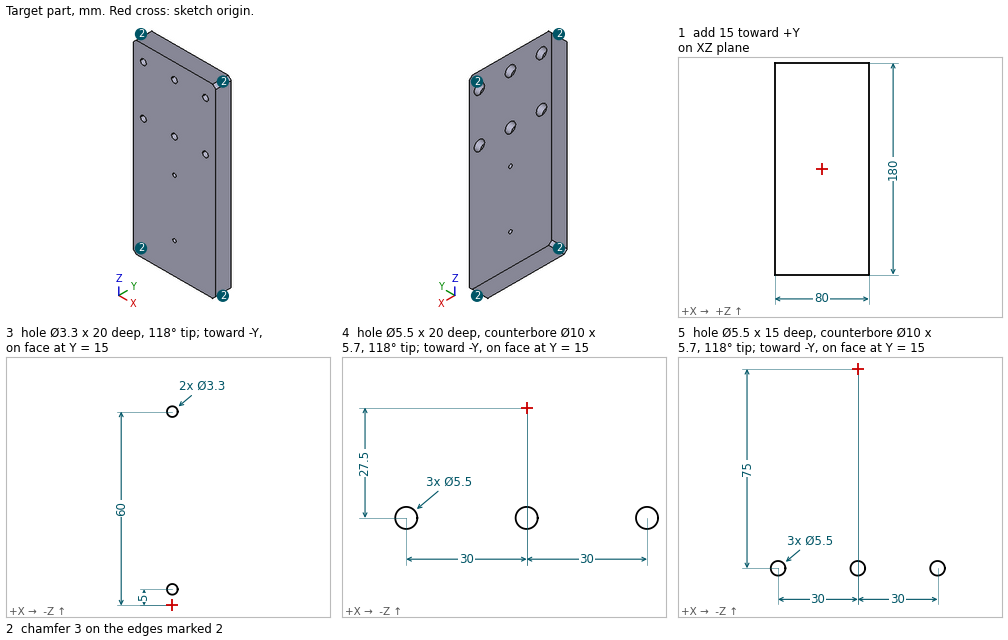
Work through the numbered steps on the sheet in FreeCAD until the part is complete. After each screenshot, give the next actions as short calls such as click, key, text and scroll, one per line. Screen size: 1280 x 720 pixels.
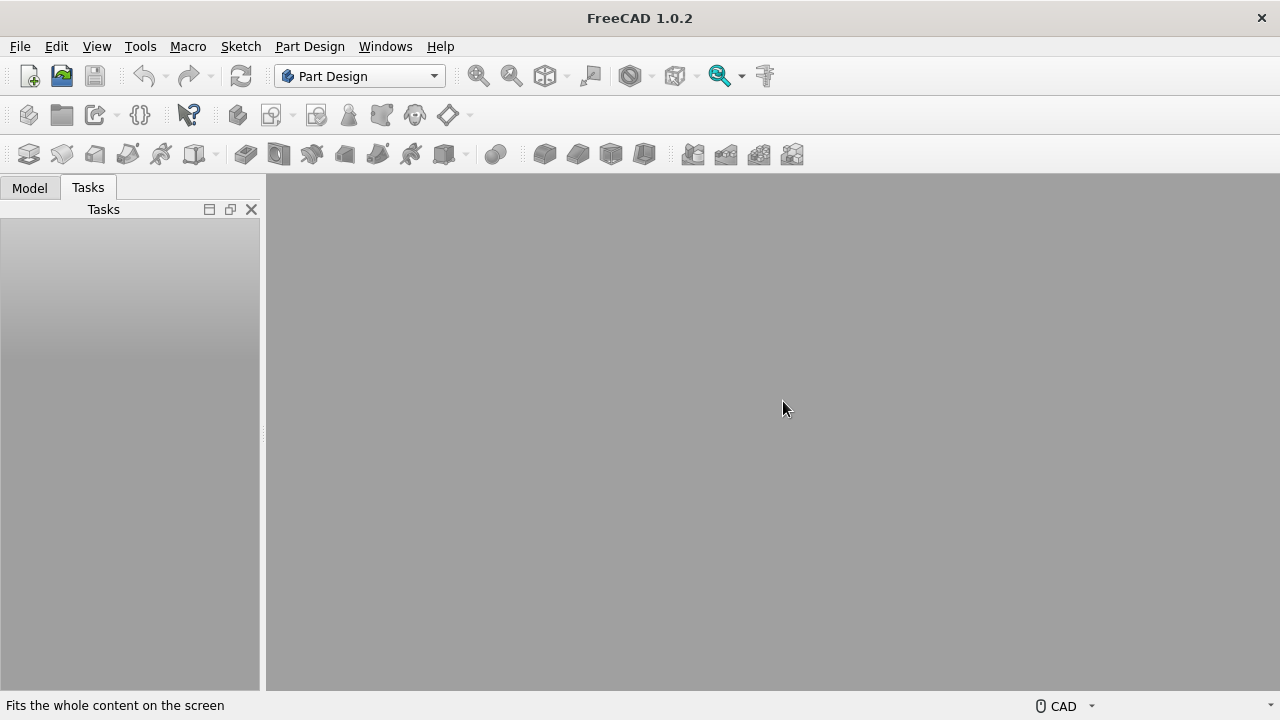
click(29, 76)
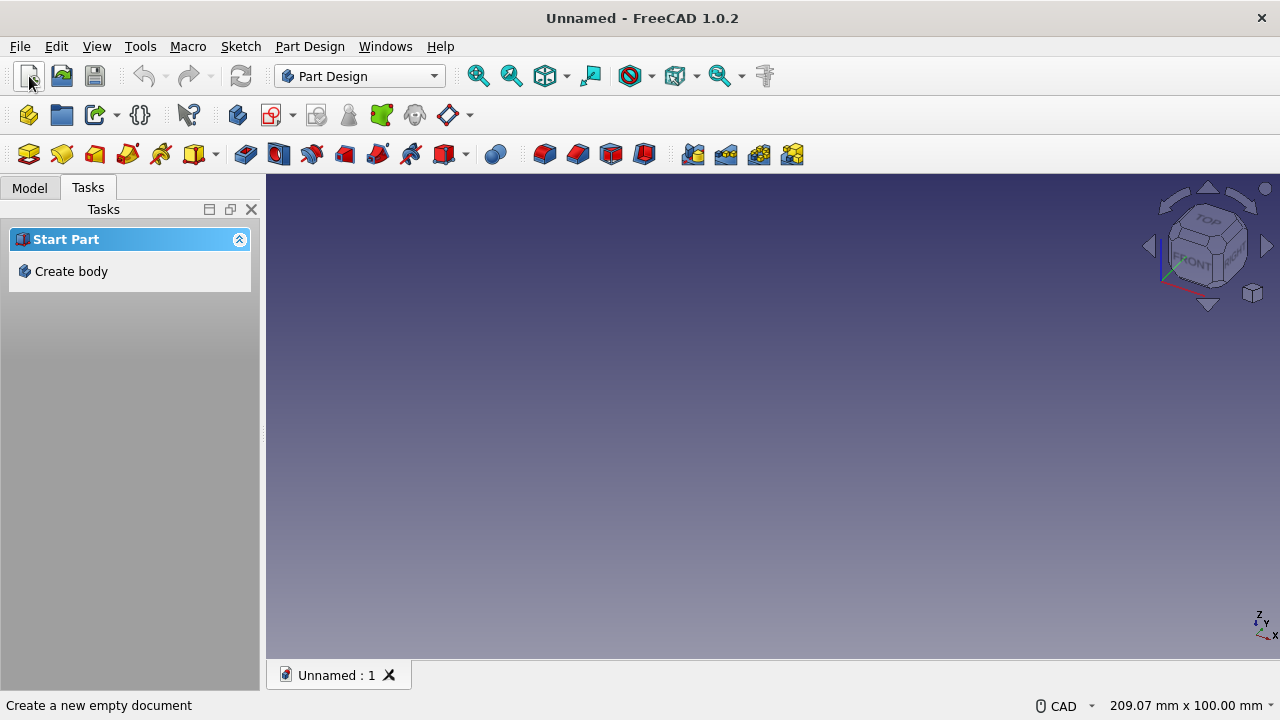
click(270, 116)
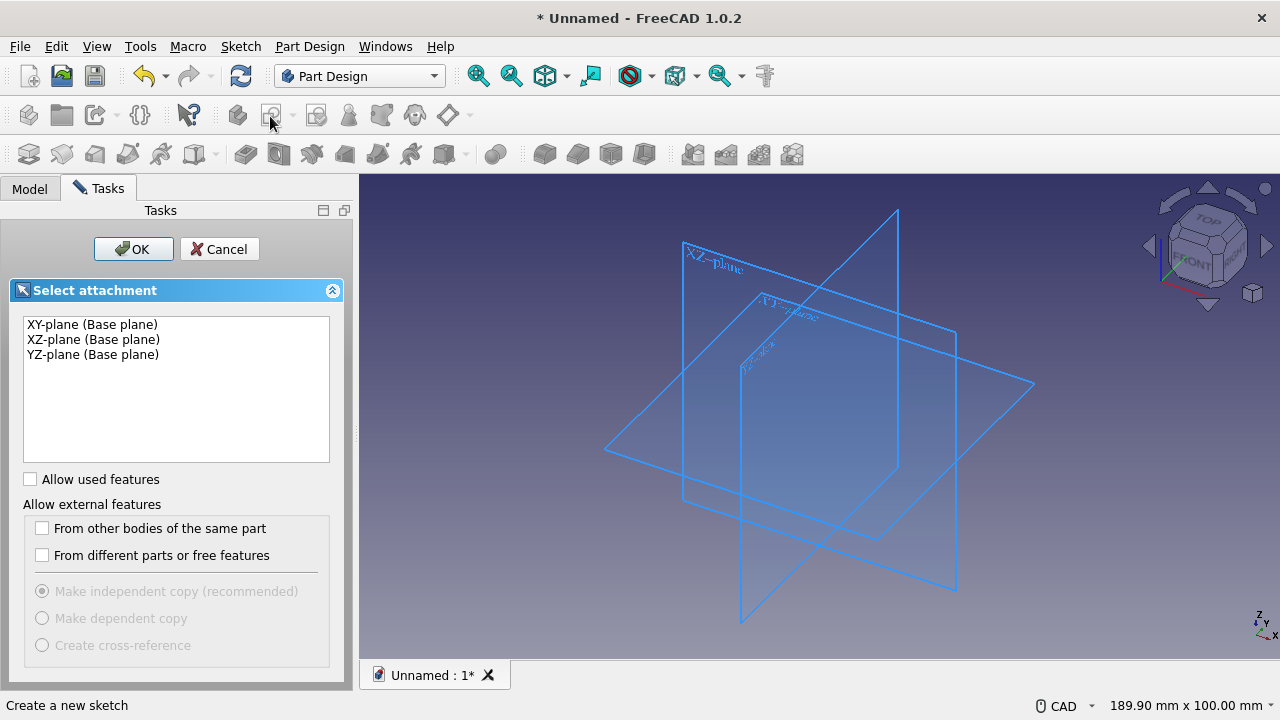
click(84, 340)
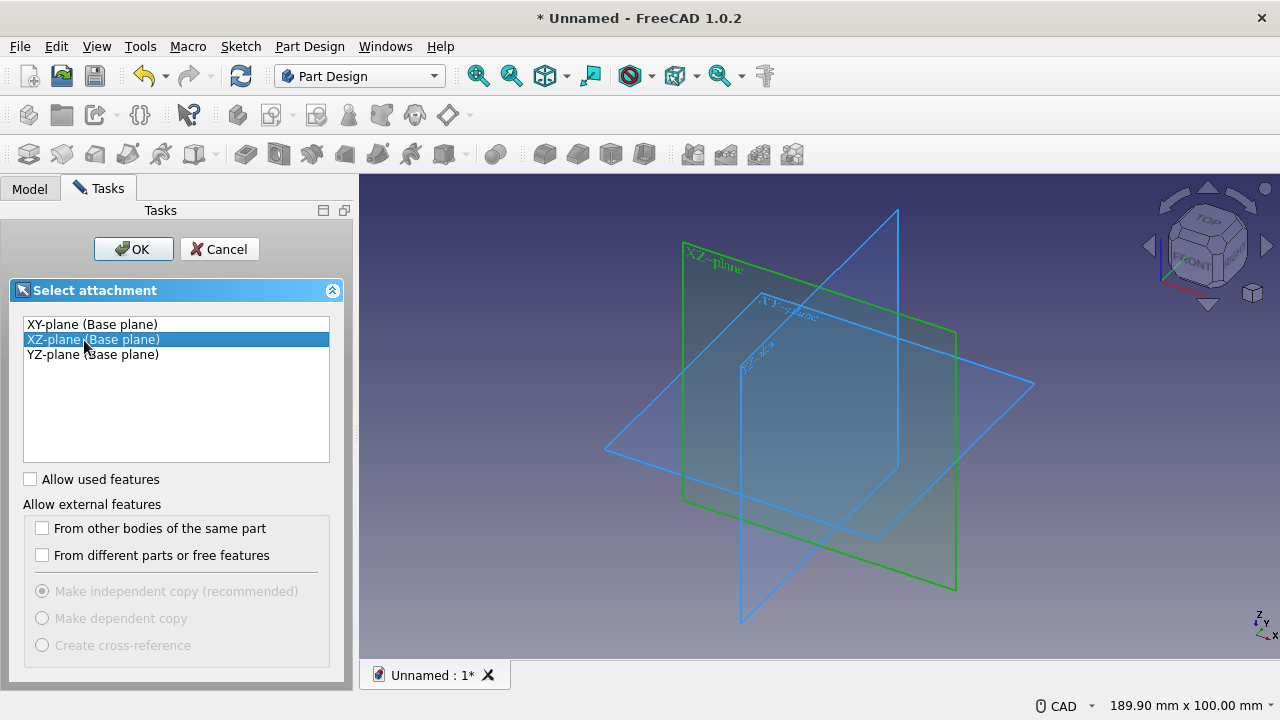
click(134, 249)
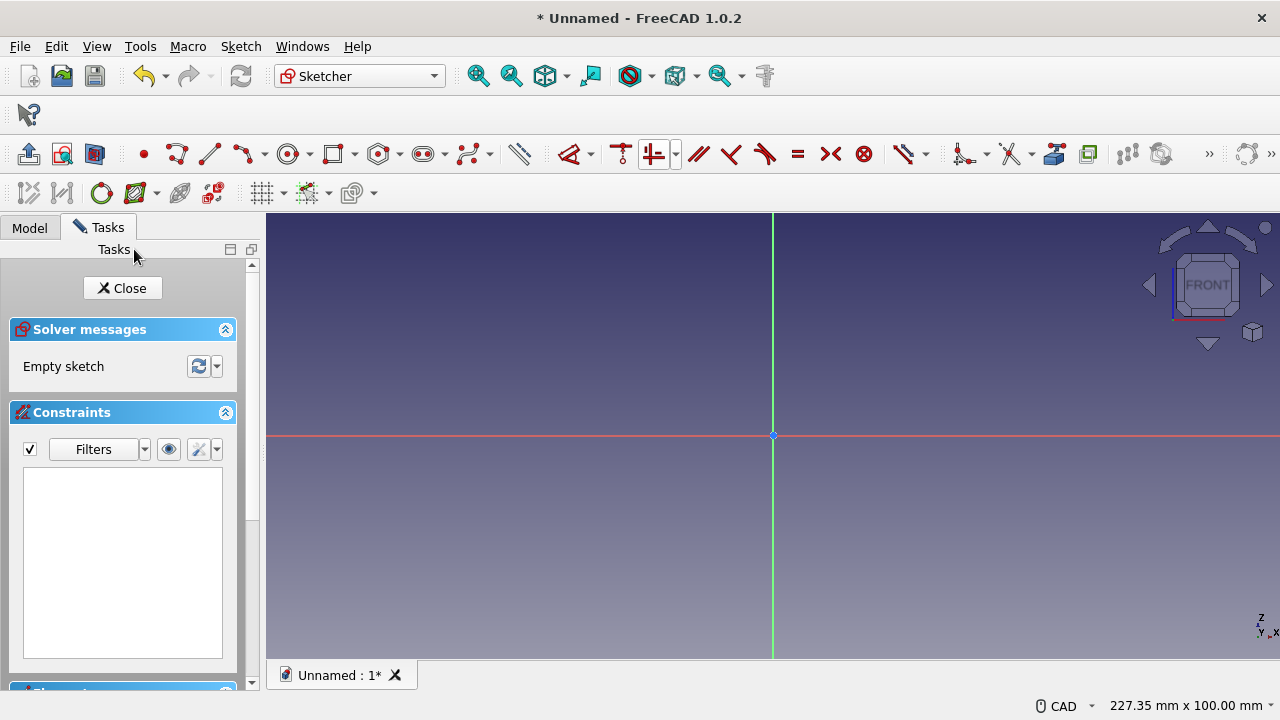
scroll(665, 436, down, 5)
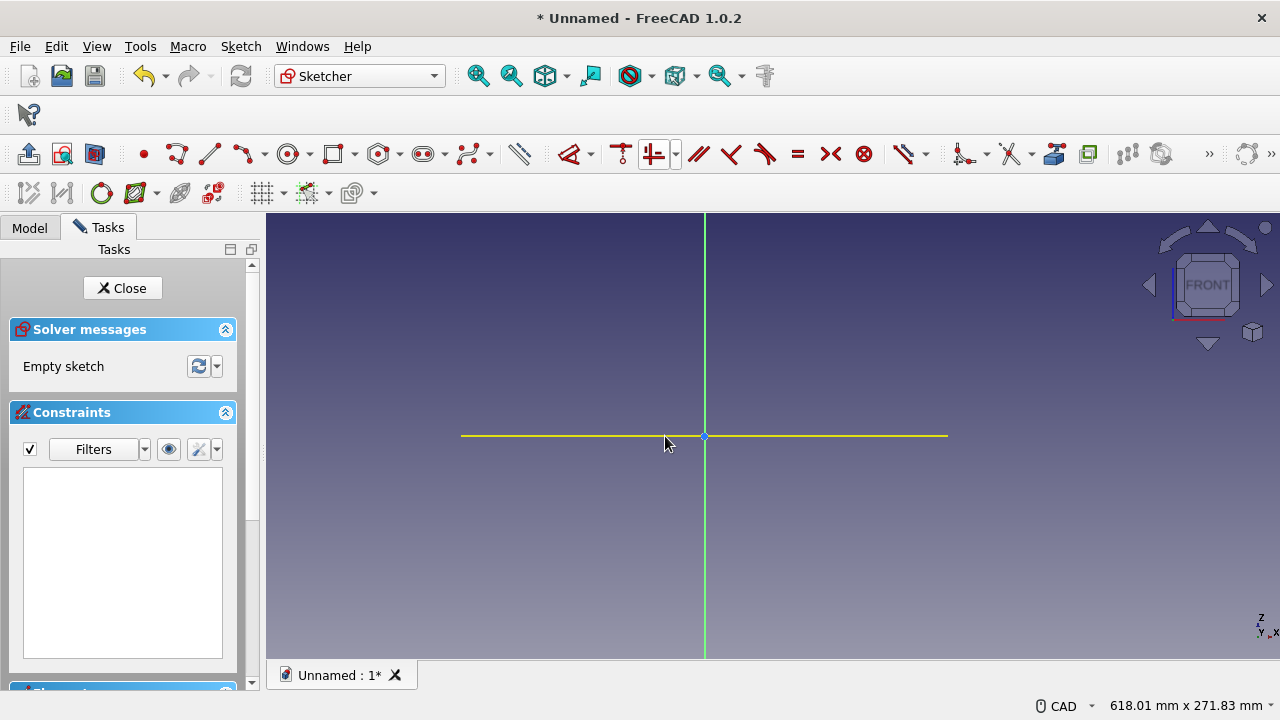
click(354, 154)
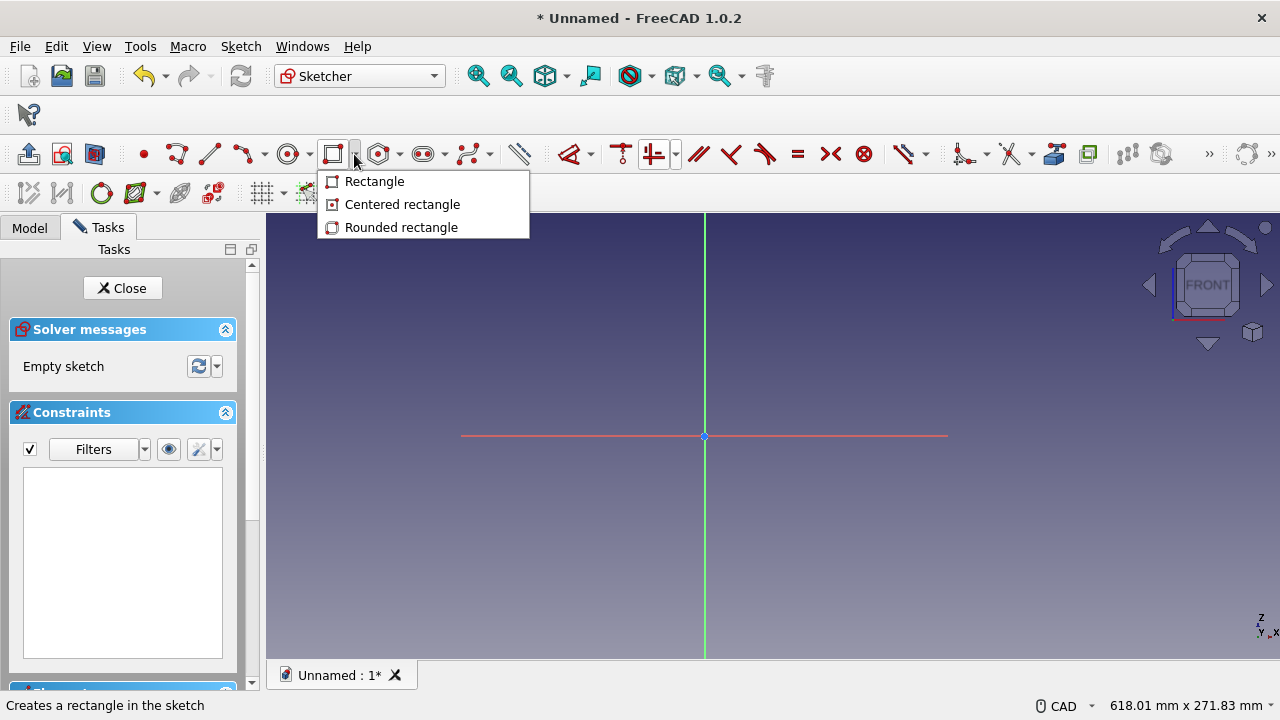
click(424, 204)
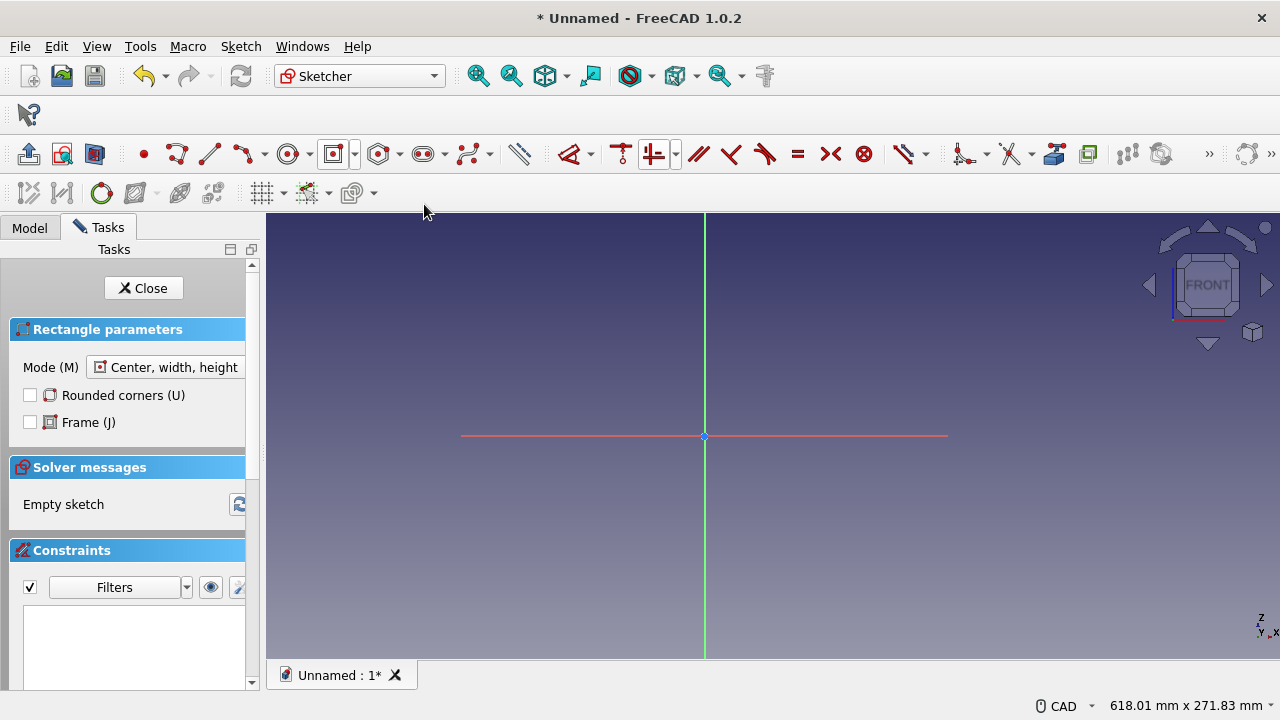
click(705, 436)
click(771, 289)
key(Escape)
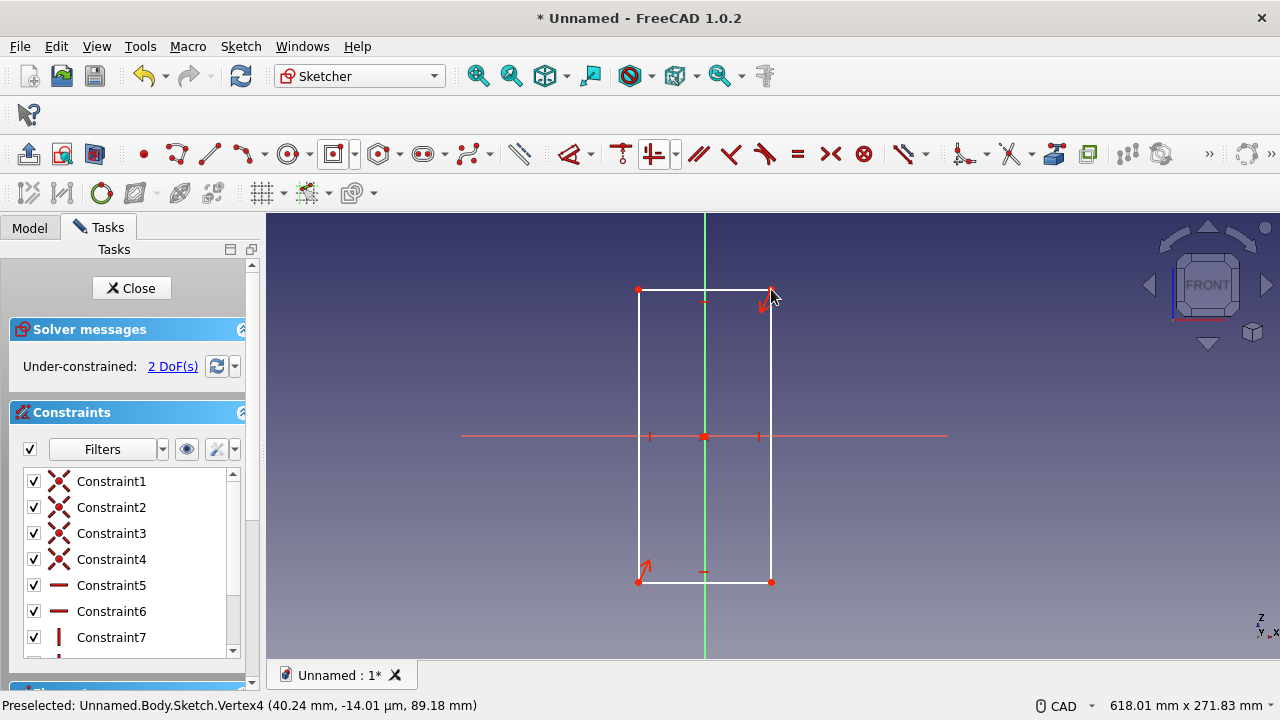
click(568, 154)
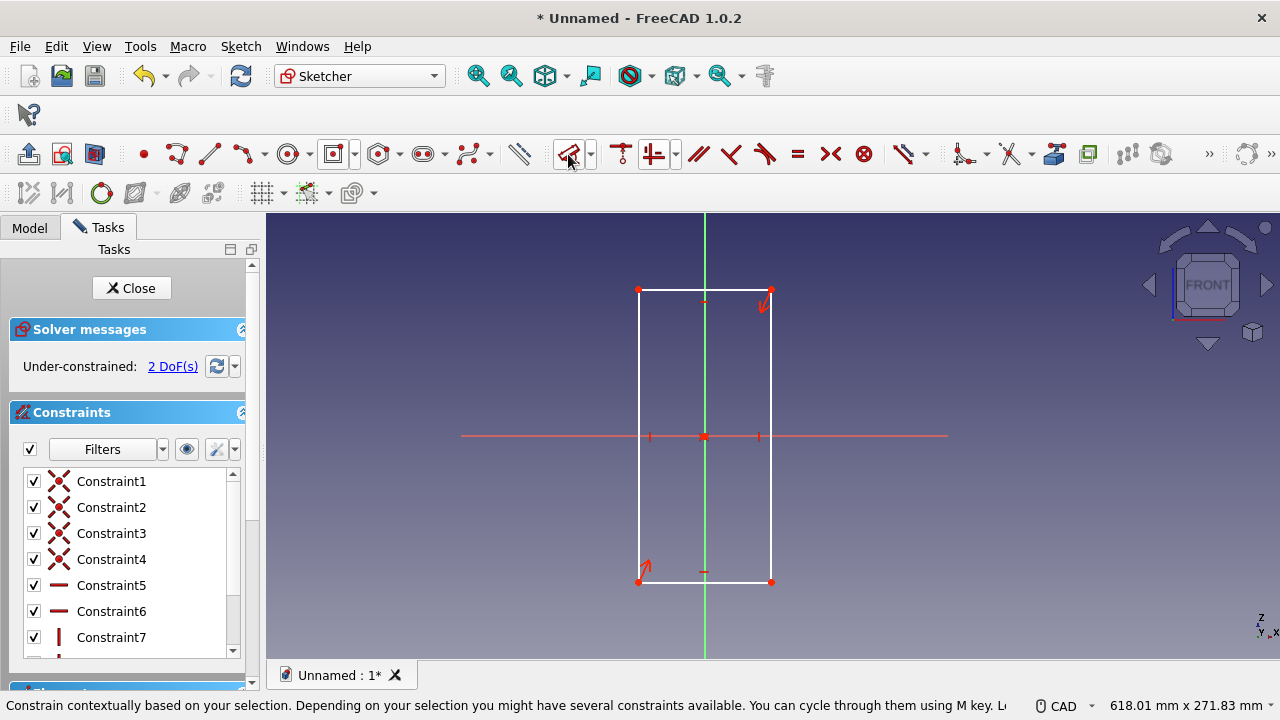
click(679, 583)
click(675, 617)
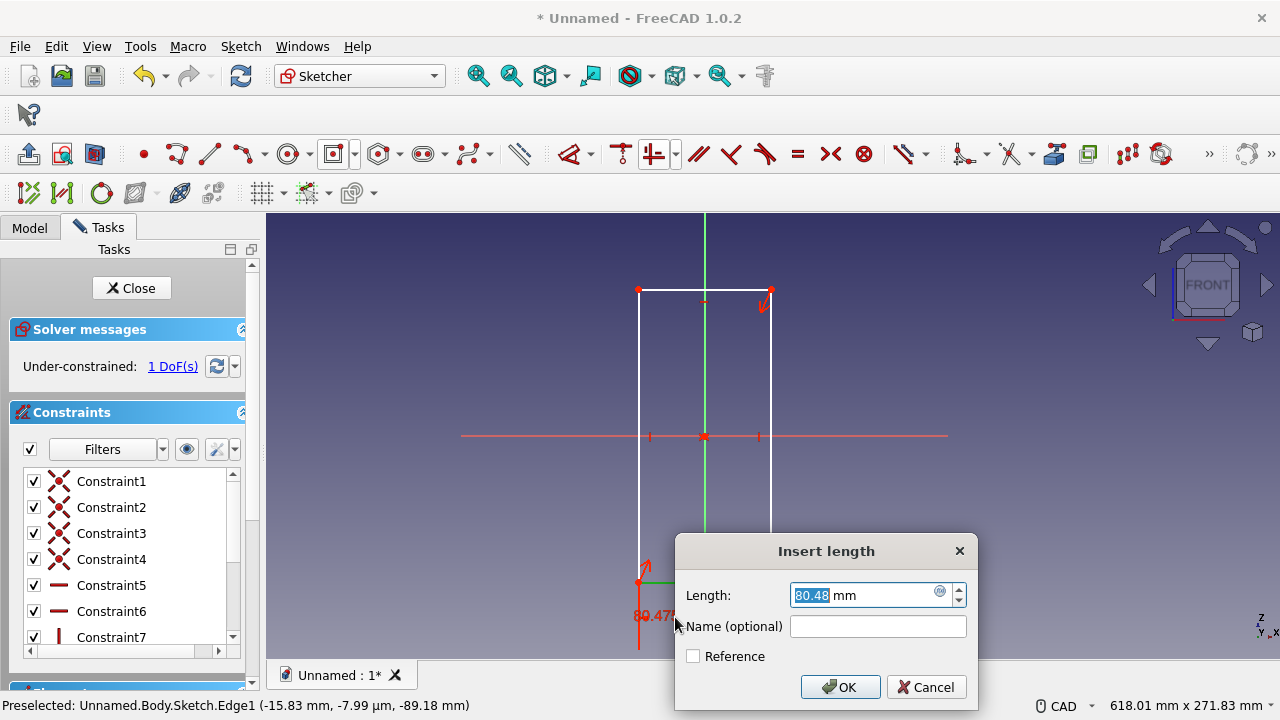
text(80)
key(Return)